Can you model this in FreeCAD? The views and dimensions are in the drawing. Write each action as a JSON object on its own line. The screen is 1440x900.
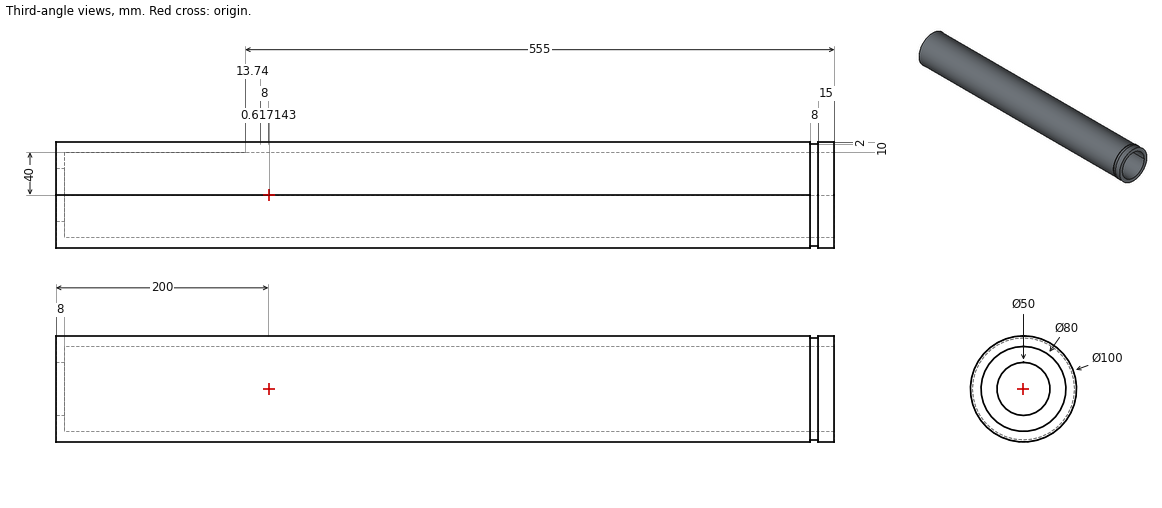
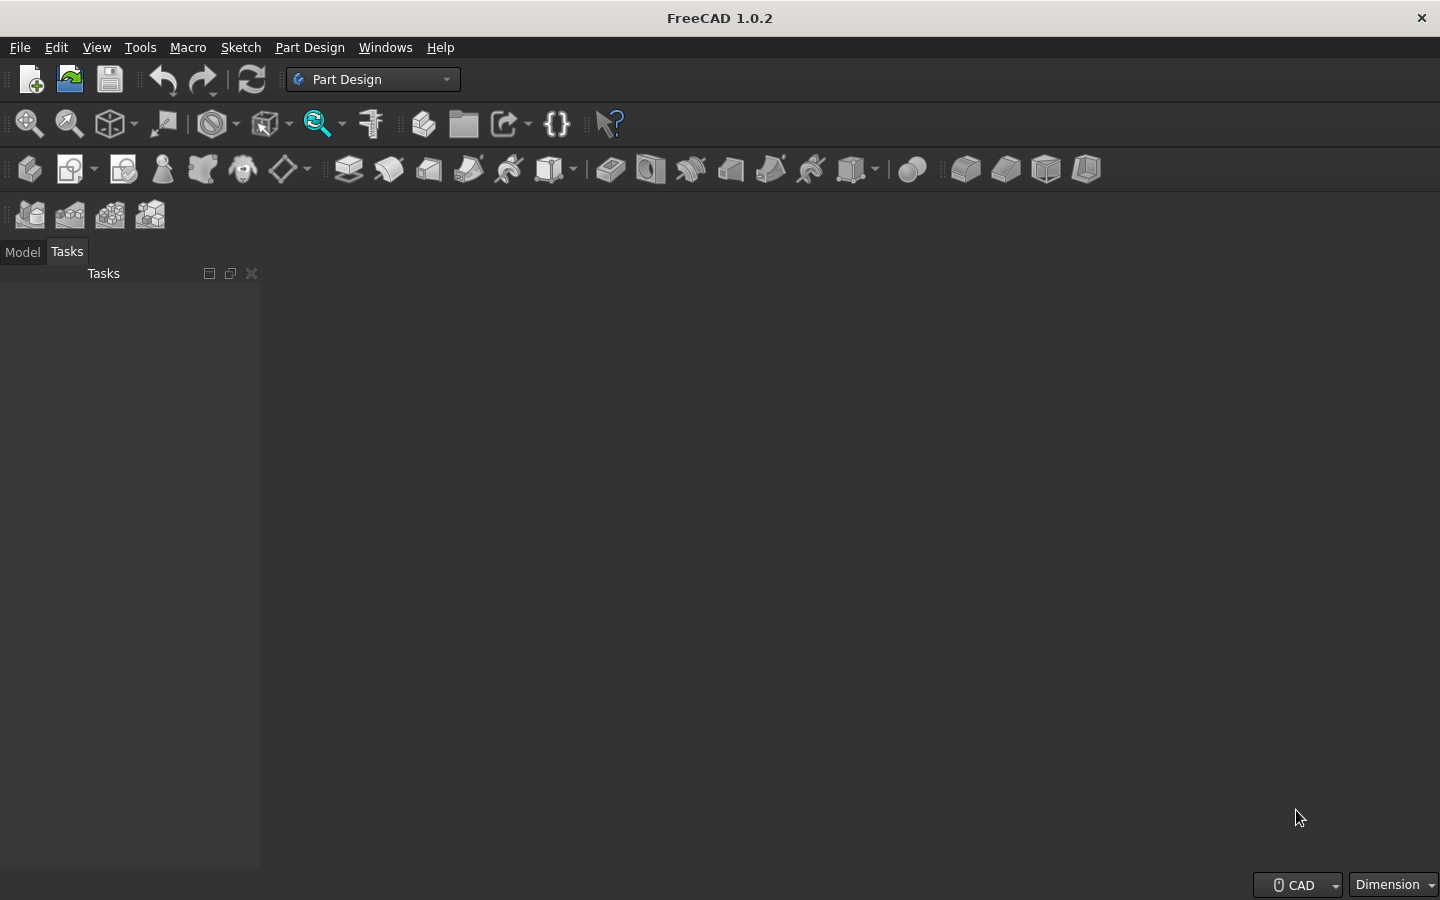
{"action": "left_click", "coordinate": [30, 80]}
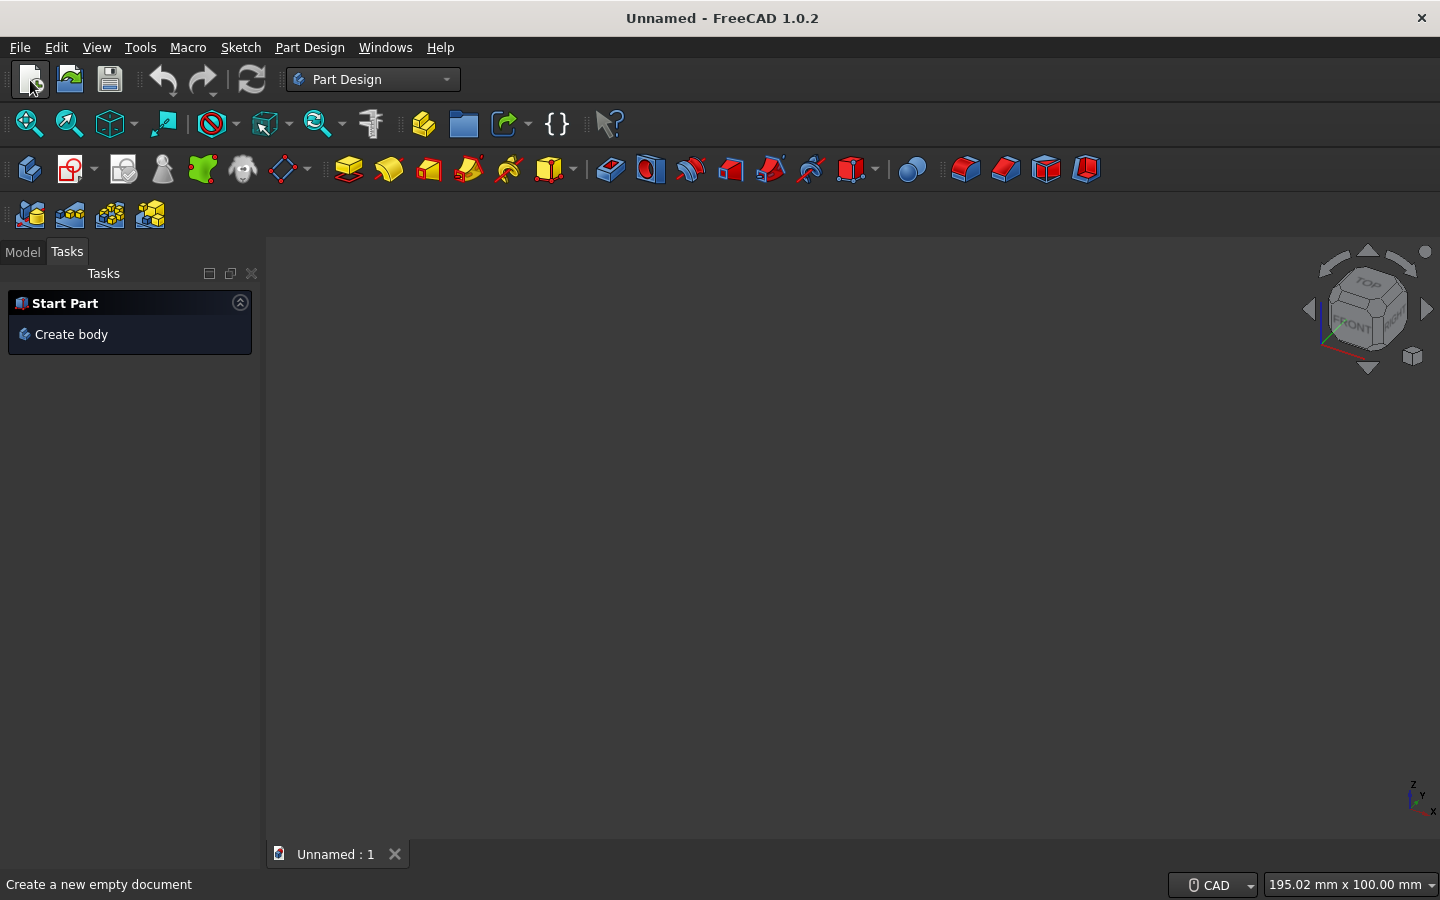
{"action": "left_click", "coordinate": [70, 170]}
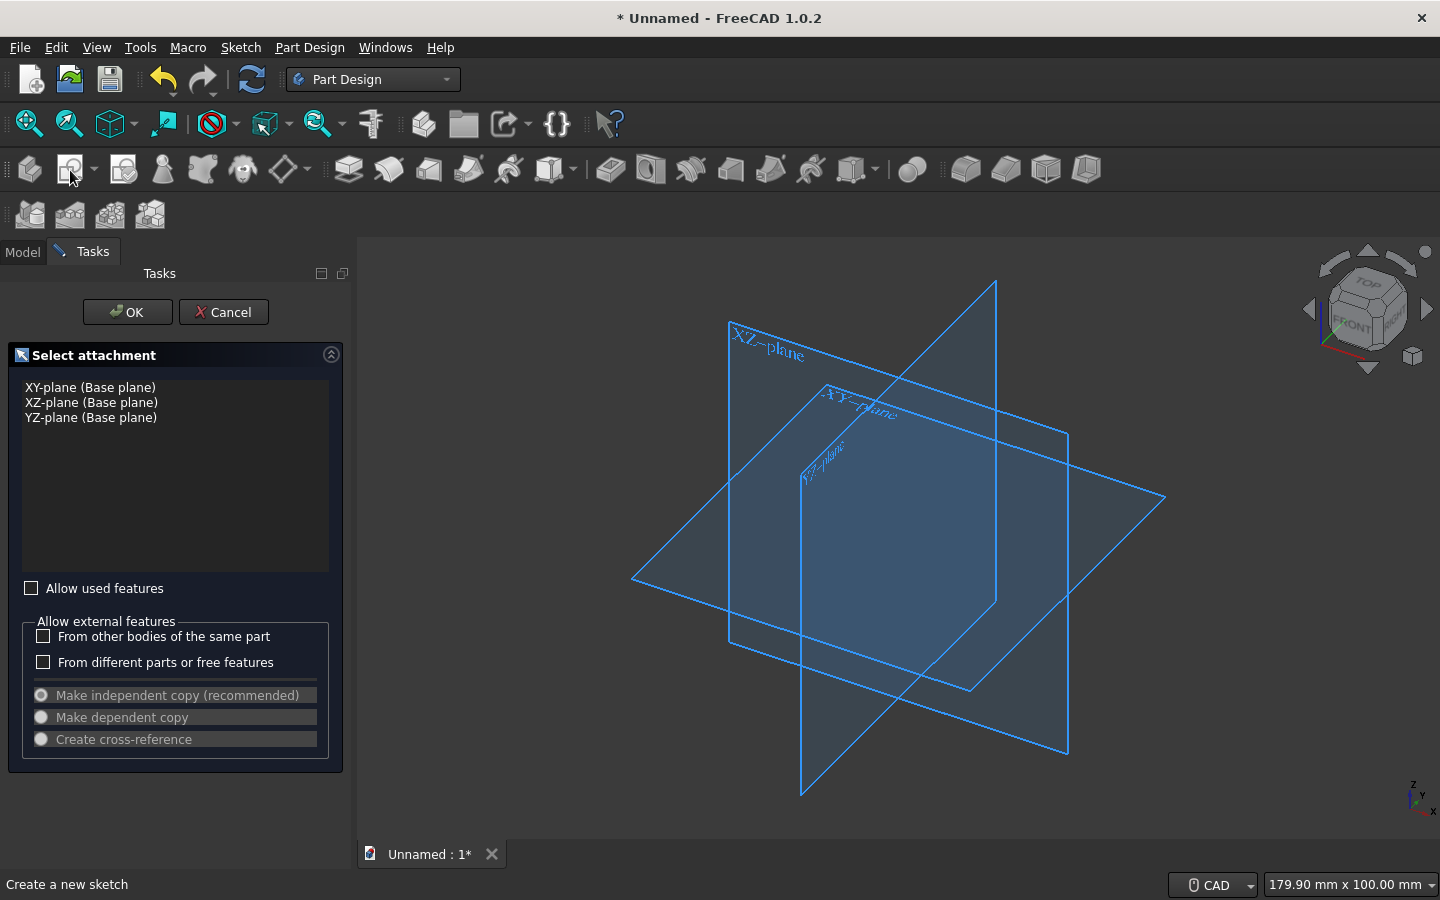
{"action": "left_click", "coordinate": [82, 388]}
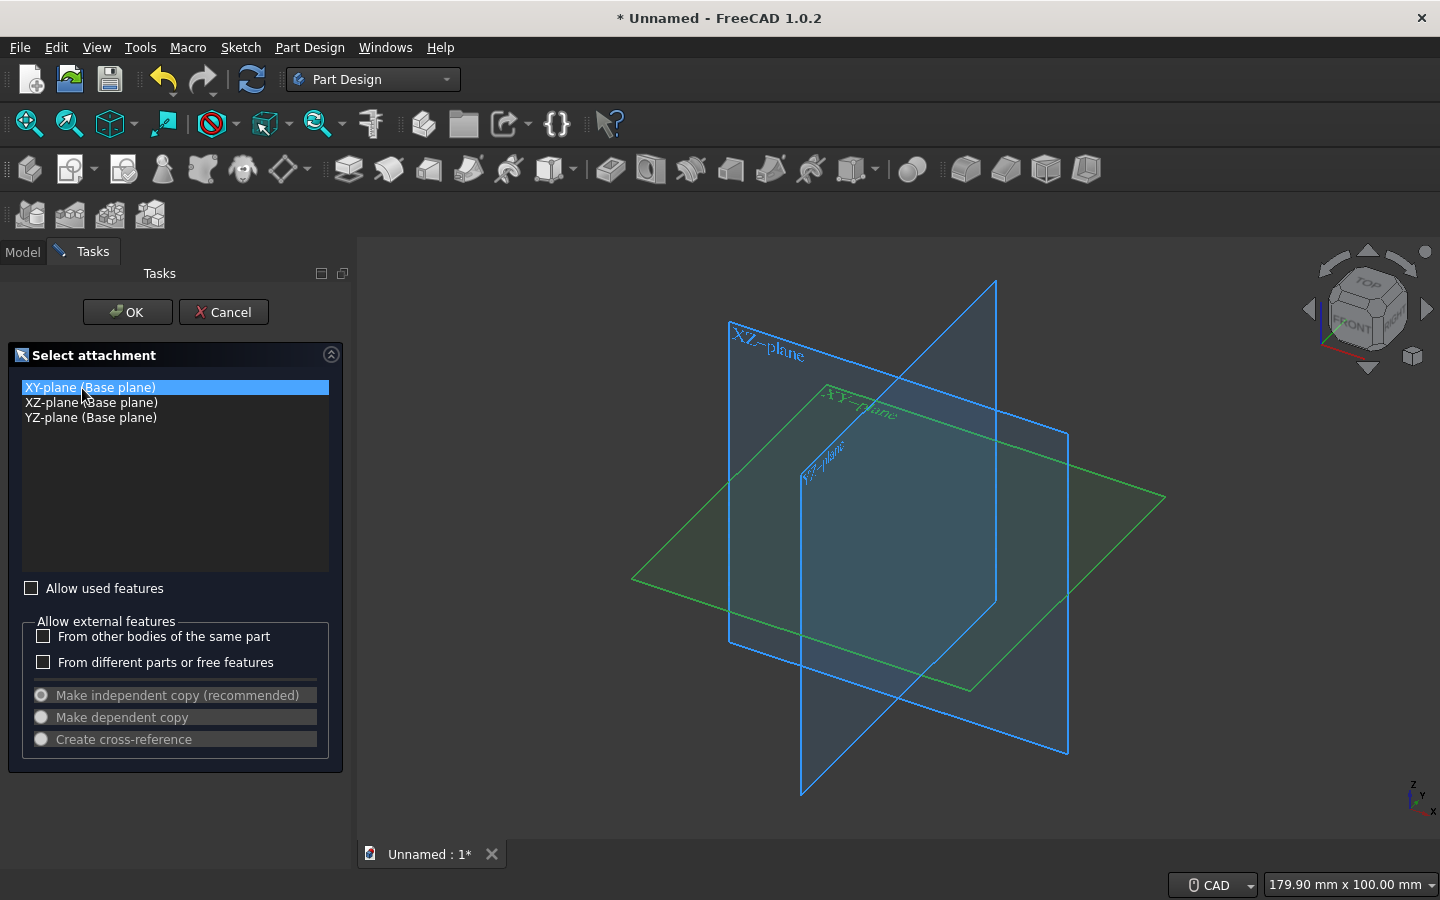
{"action": "left_click", "coordinate": [128, 312]}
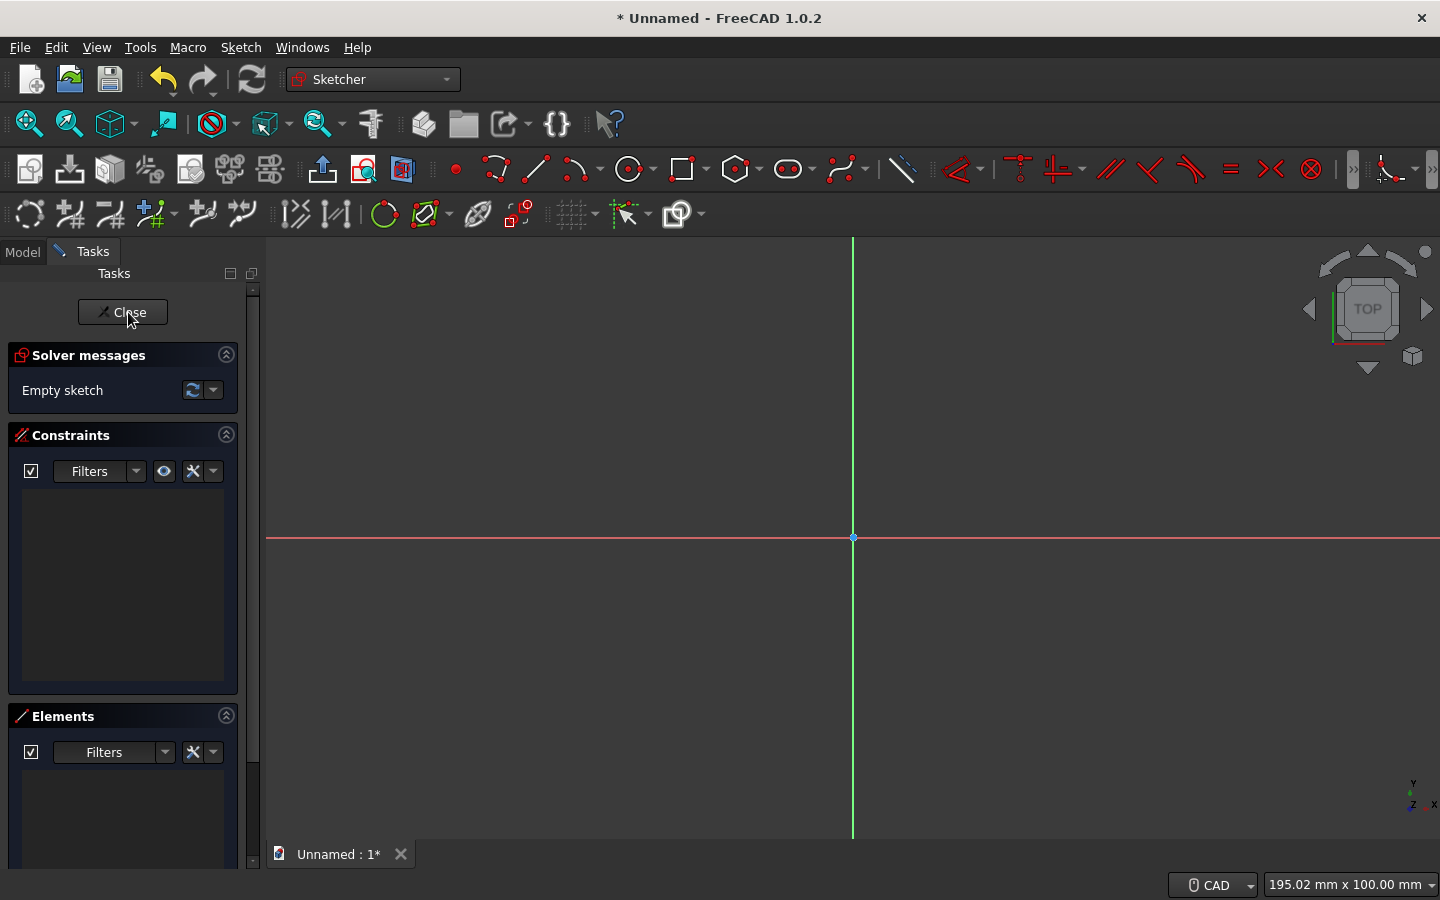
{"action": "scroll", "coordinate": [379, 576], "scroll_direction": "down", "scroll_amount": 8}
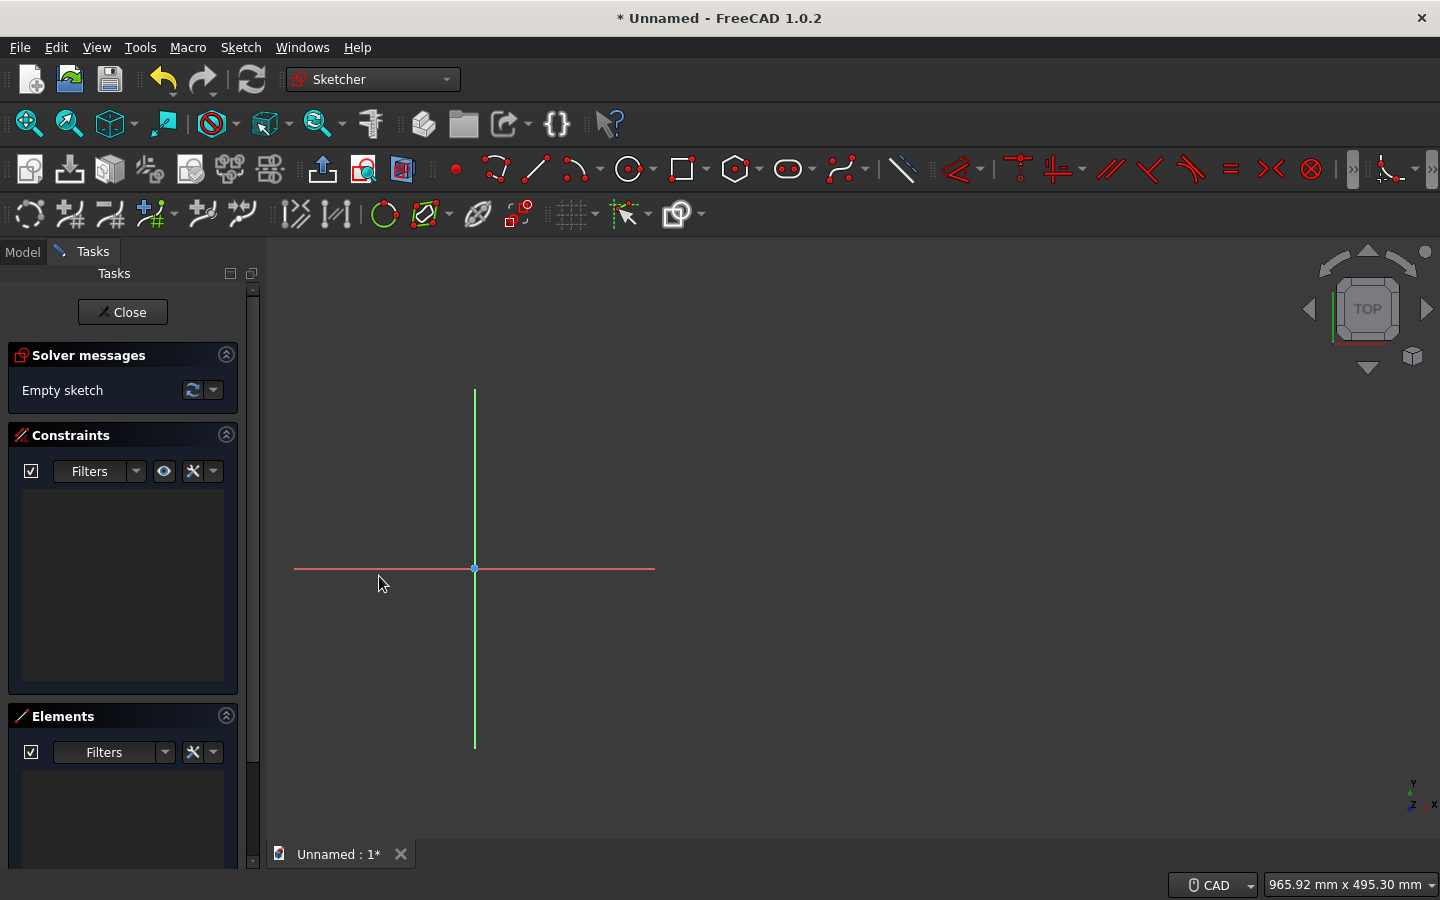
{"action": "left_click", "coordinate": [496, 170]}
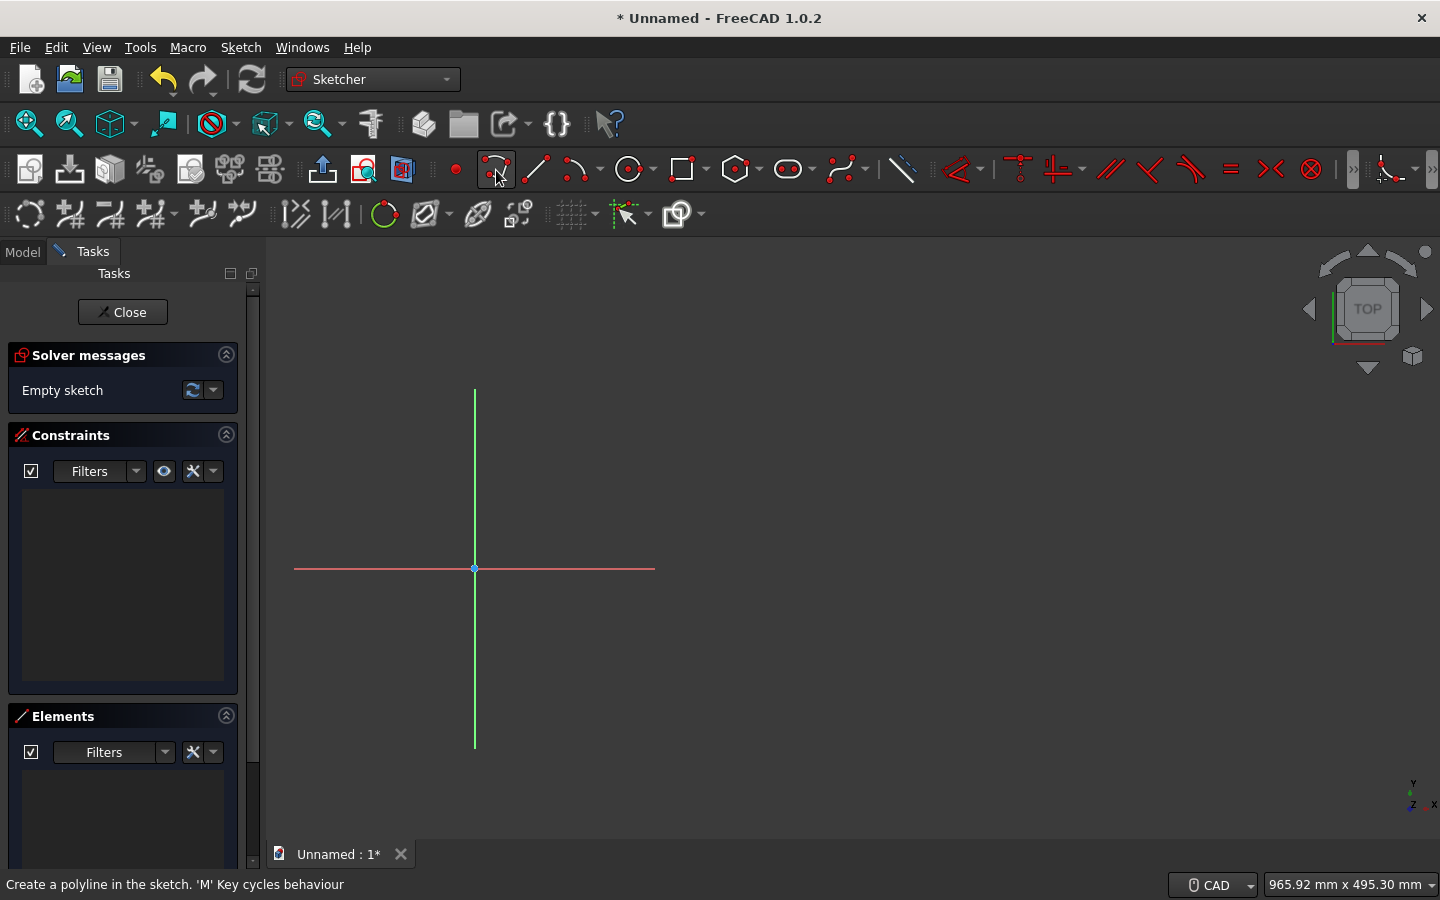
{"action": "left_click", "coordinate": [448, 520]}
{"action": "left_click", "coordinate": [1122, 520]}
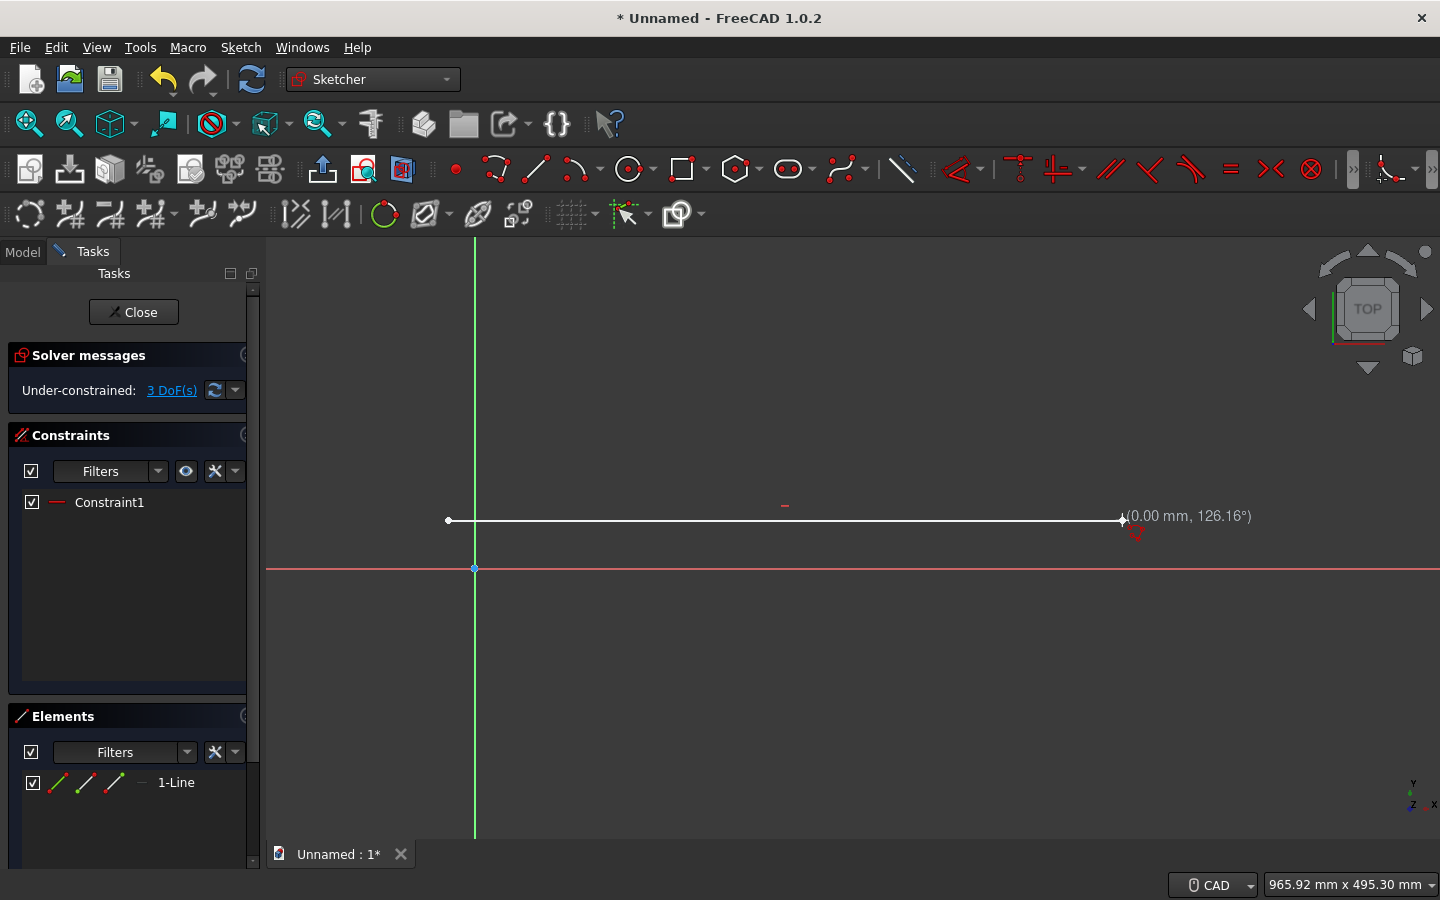
{"action": "scroll", "coordinate": [1122, 508], "scroll_direction": "up", "scroll_amount": 2}